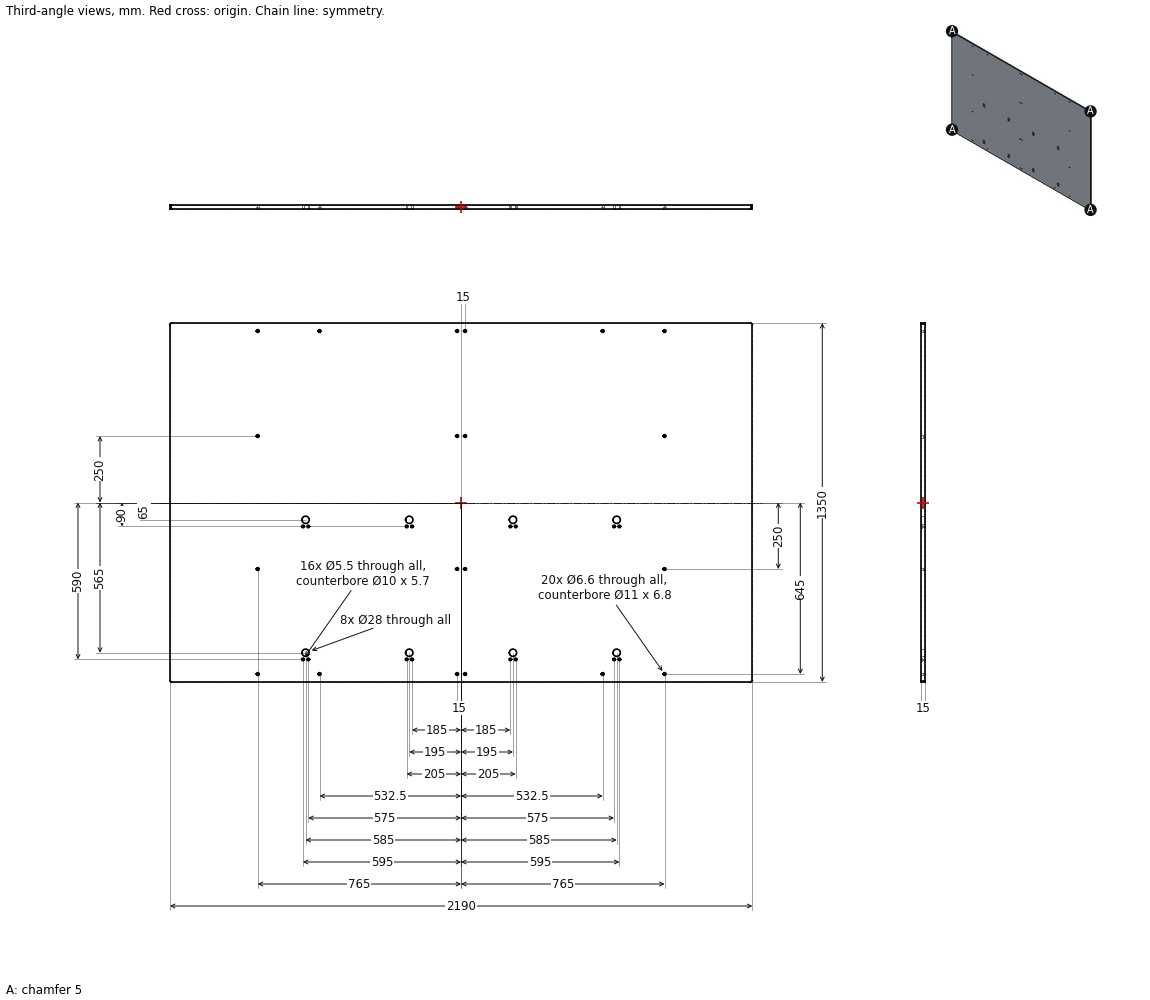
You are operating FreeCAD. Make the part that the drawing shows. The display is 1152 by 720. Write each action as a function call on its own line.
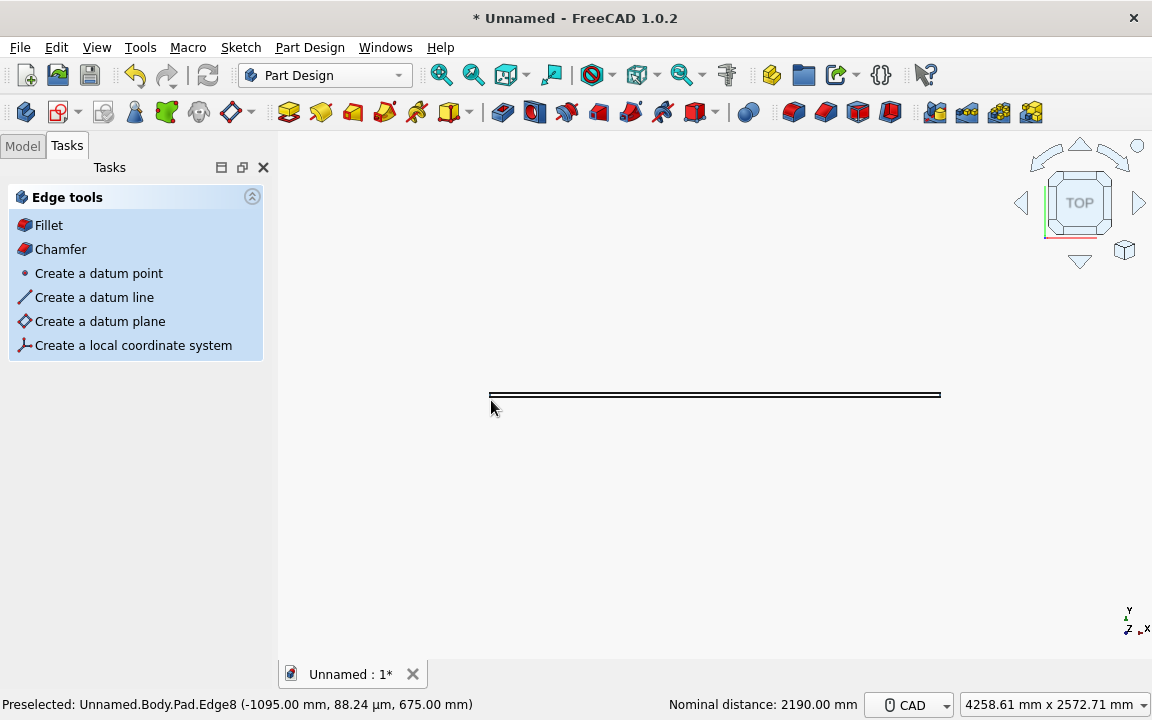
key(1)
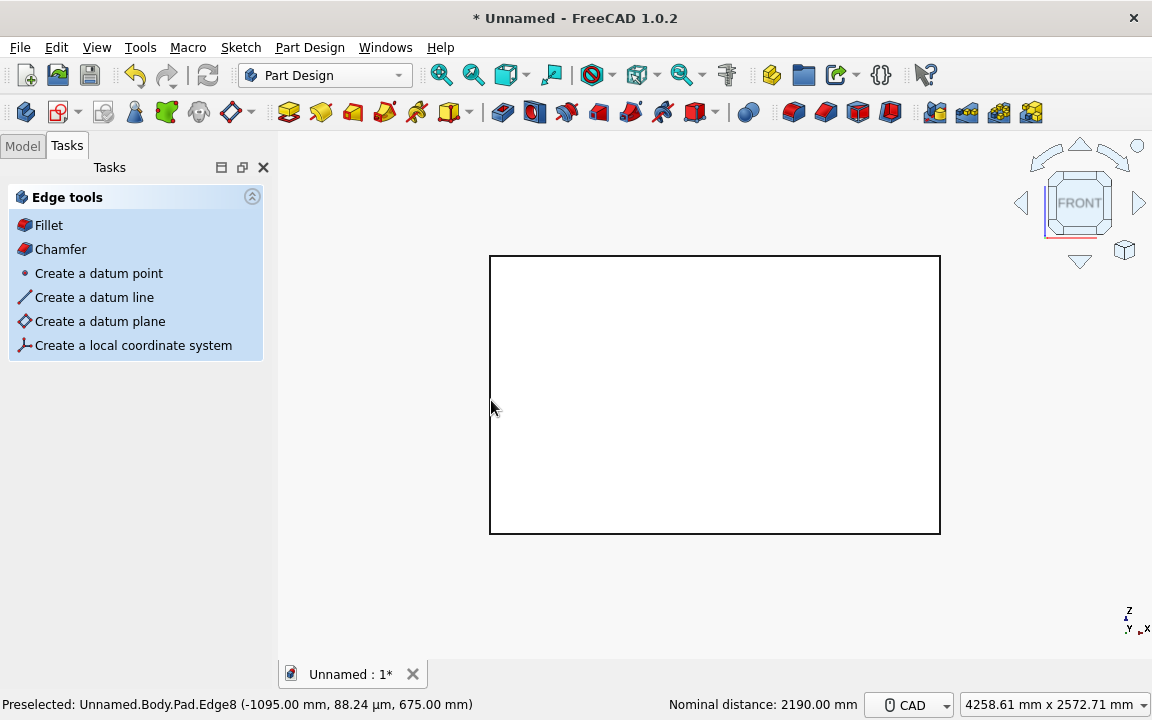
scroll(490, 533, up, 13)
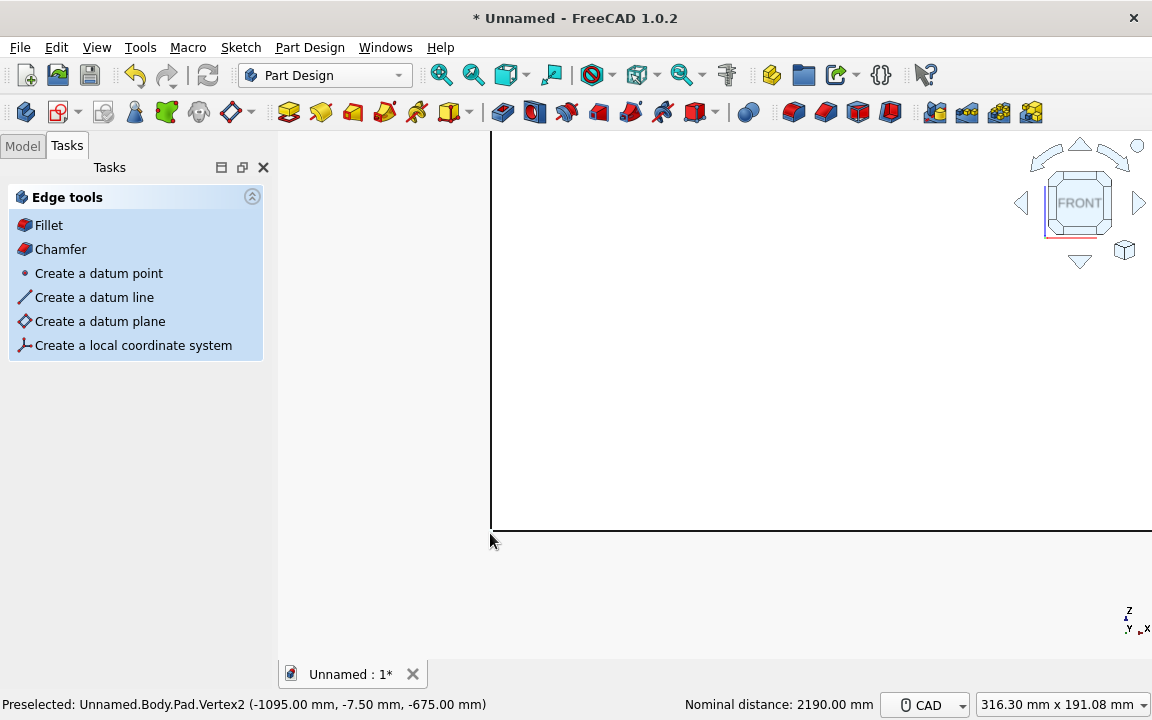
key(v)
key(f)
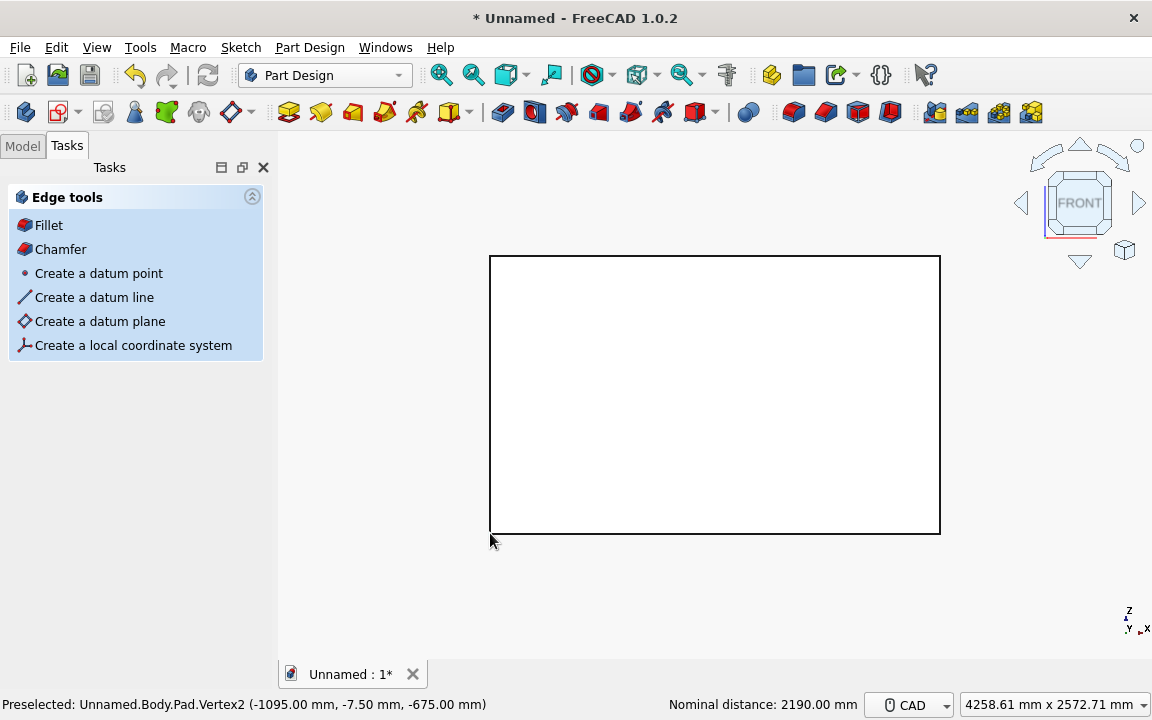
key(3)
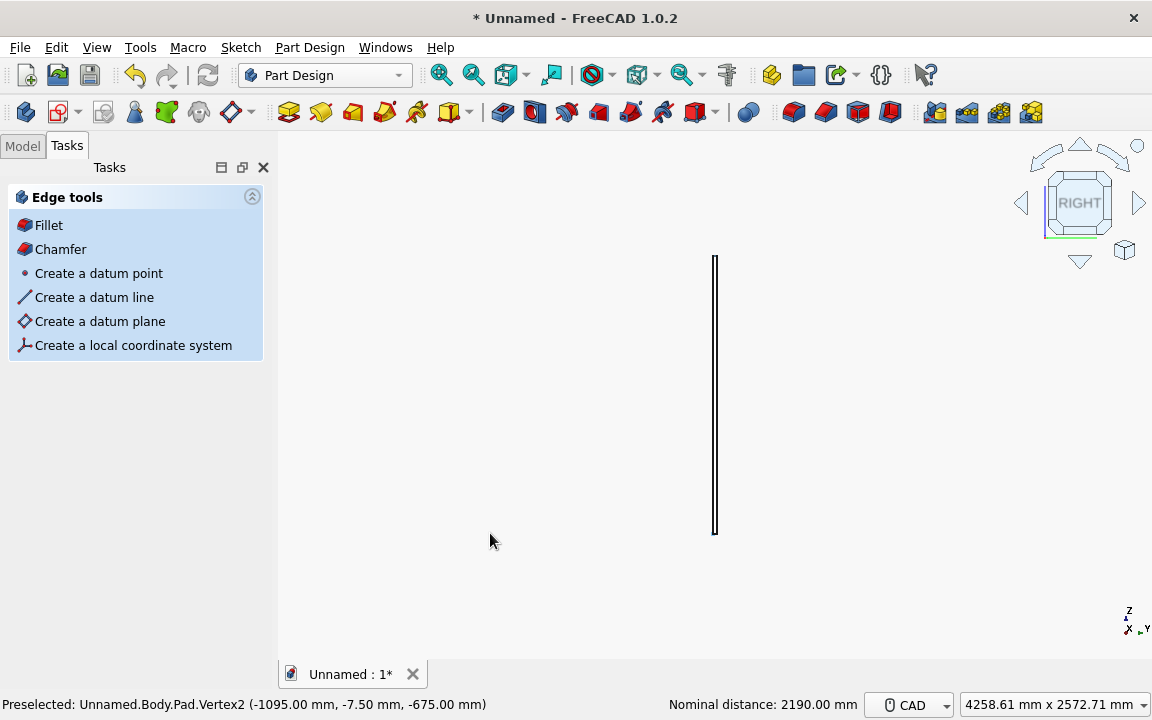
scroll(715, 533, up, 13)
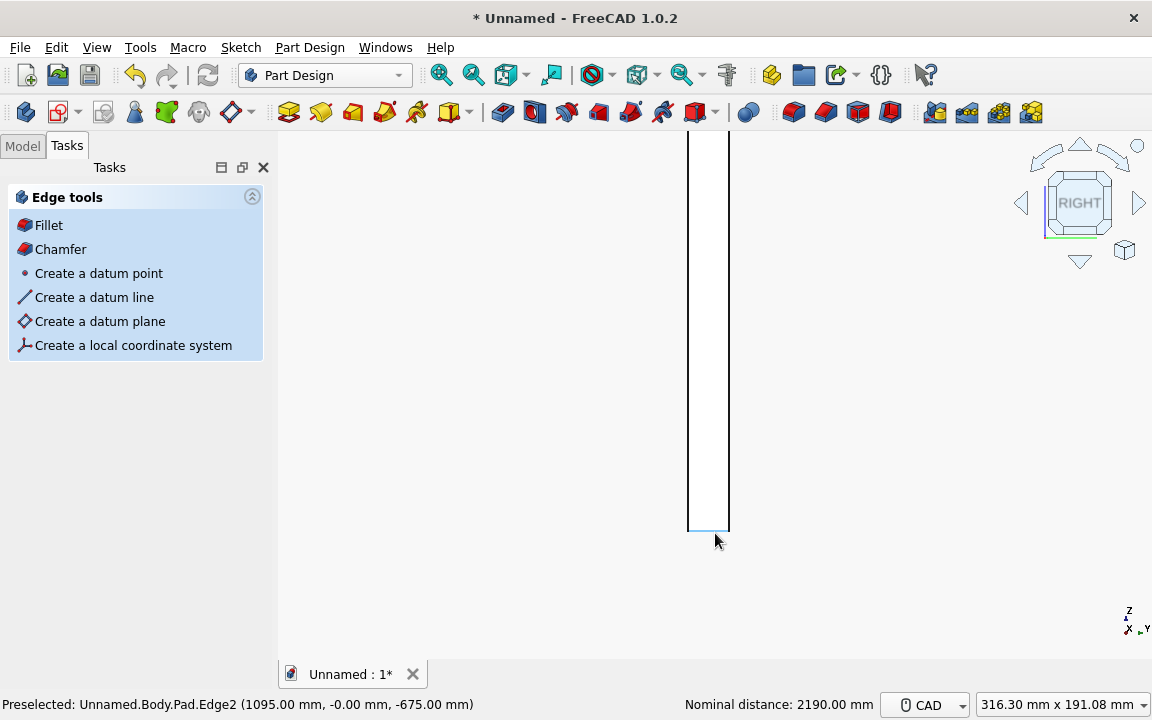
click(709, 530, ctrl)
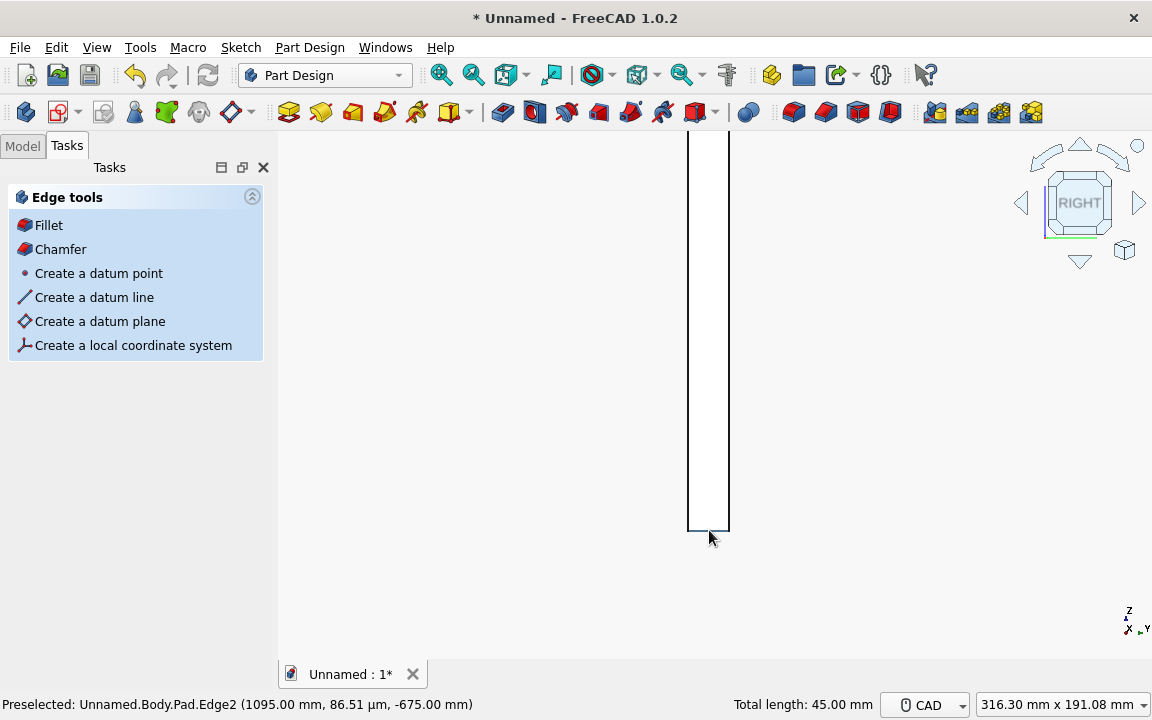
key(v)
key(f)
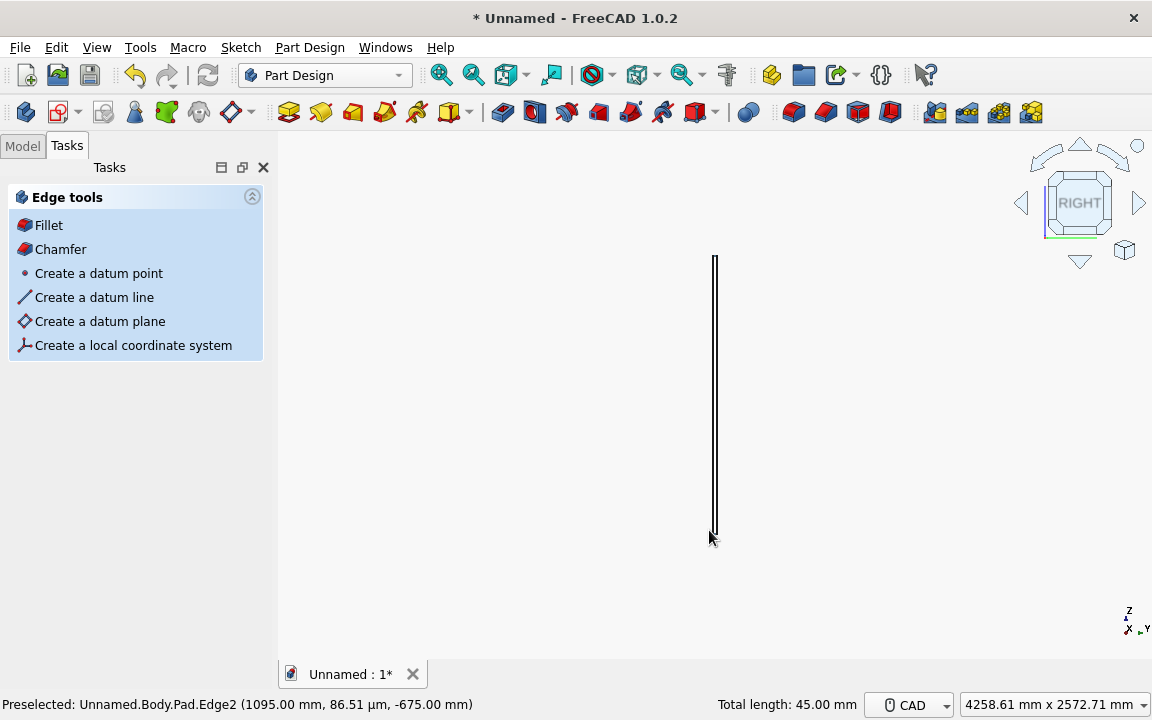
key(5)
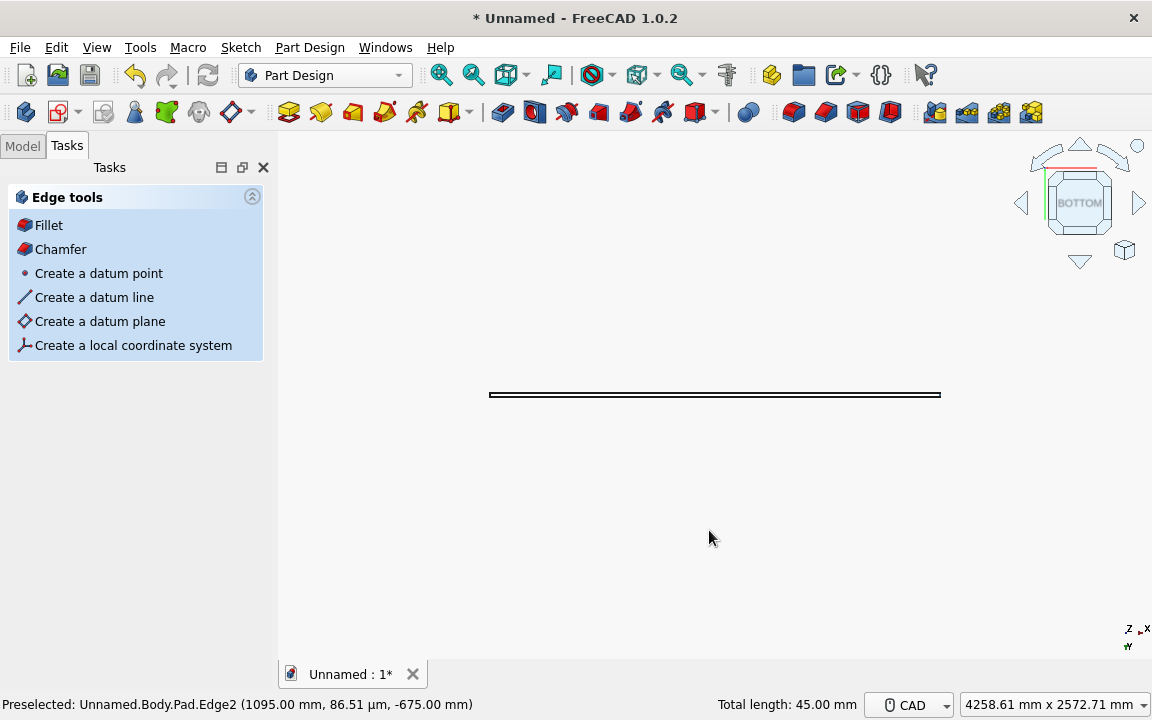
scroll(490, 394, up, 13)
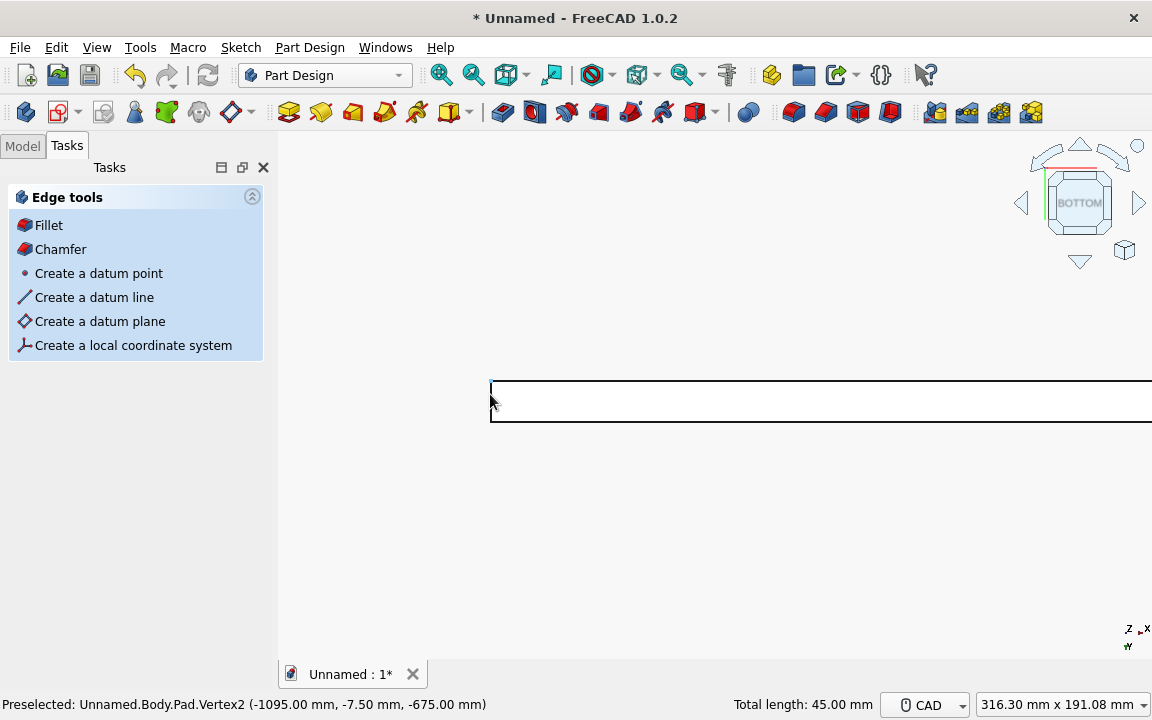
click(491, 400, ctrl)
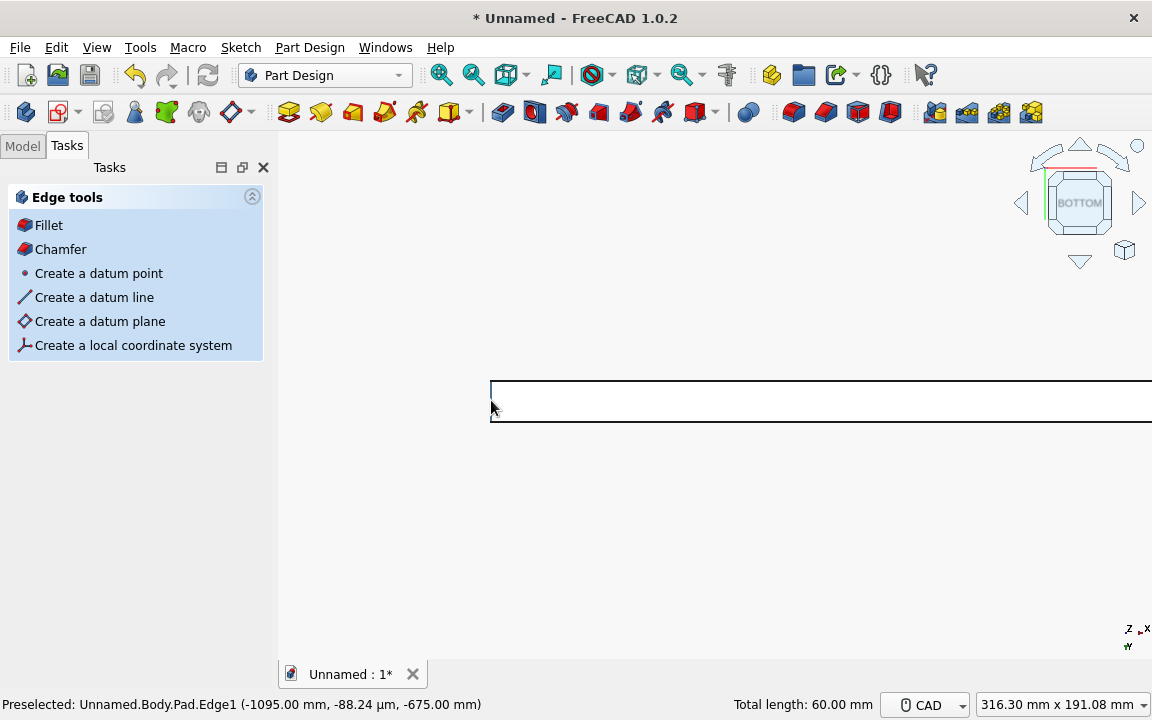
click(826, 112)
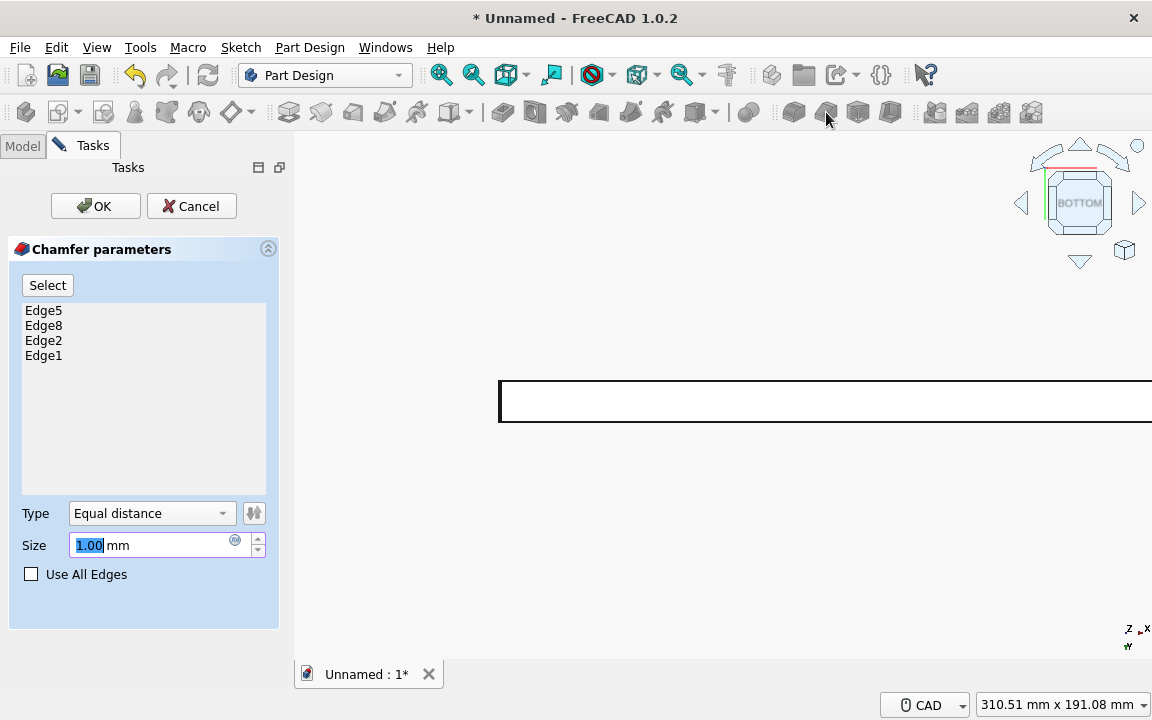
text(5)
key(Tab)